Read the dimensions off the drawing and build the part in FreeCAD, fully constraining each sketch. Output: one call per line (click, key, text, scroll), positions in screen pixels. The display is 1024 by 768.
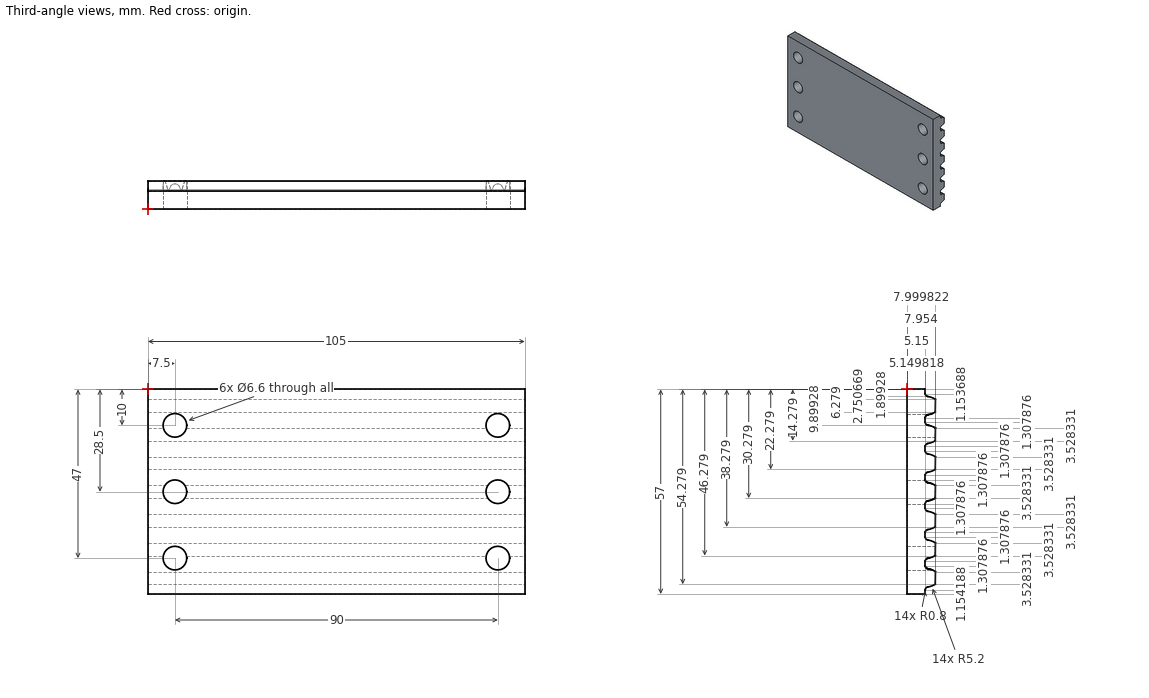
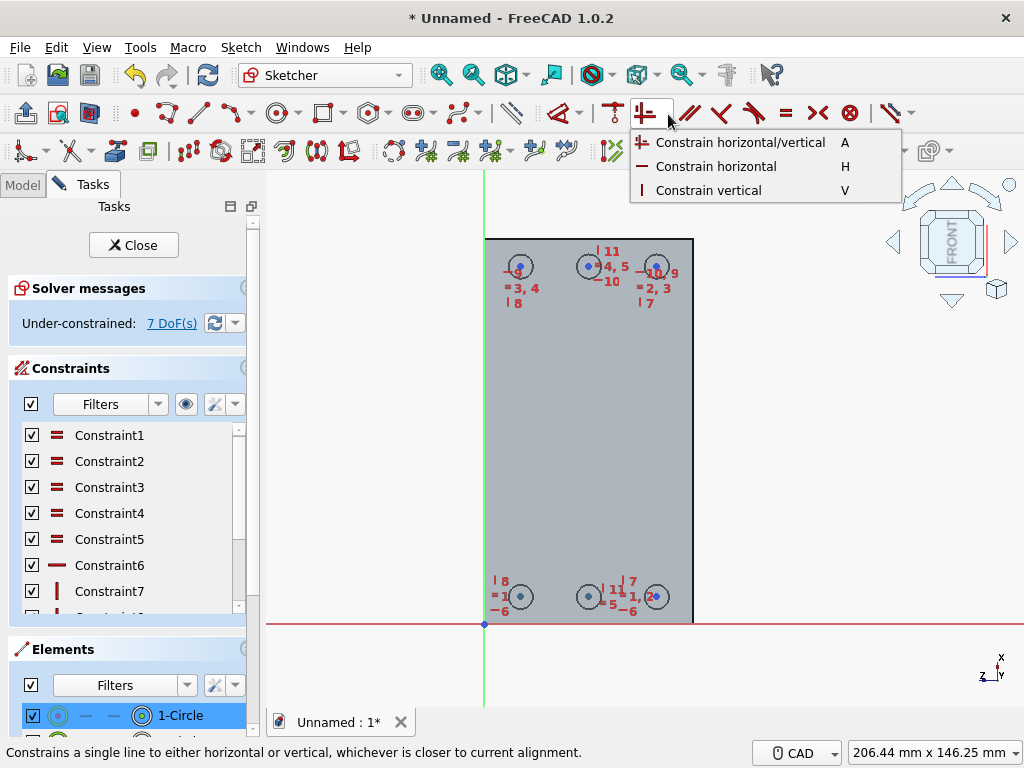
click(766, 166)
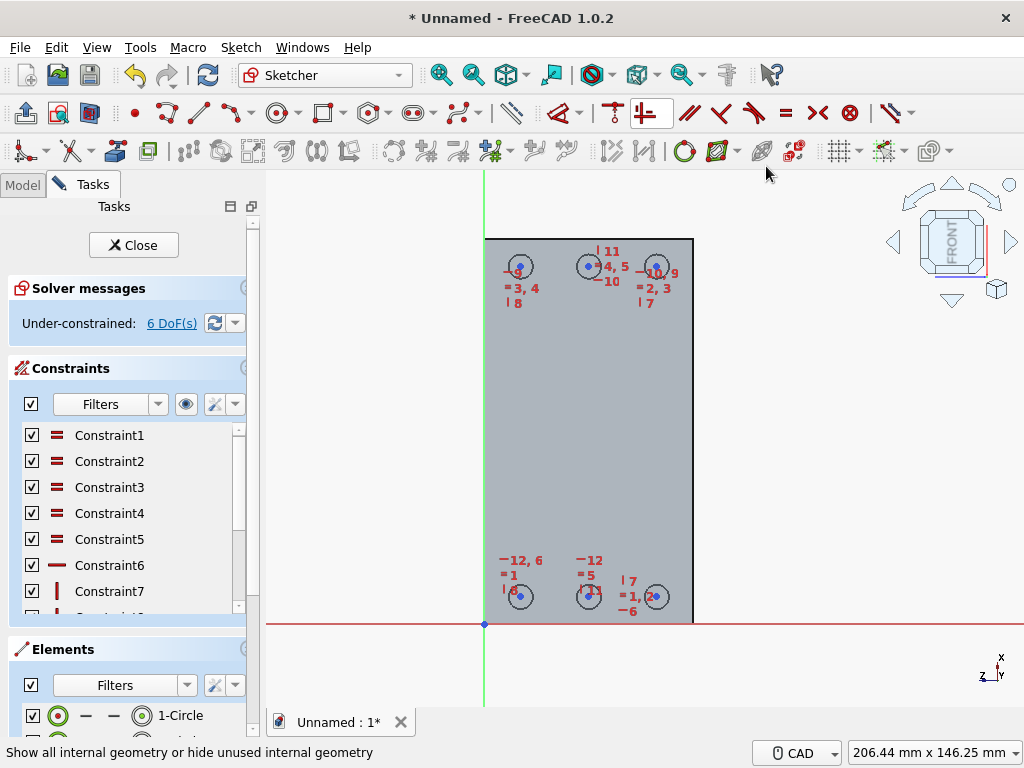
click(558, 114)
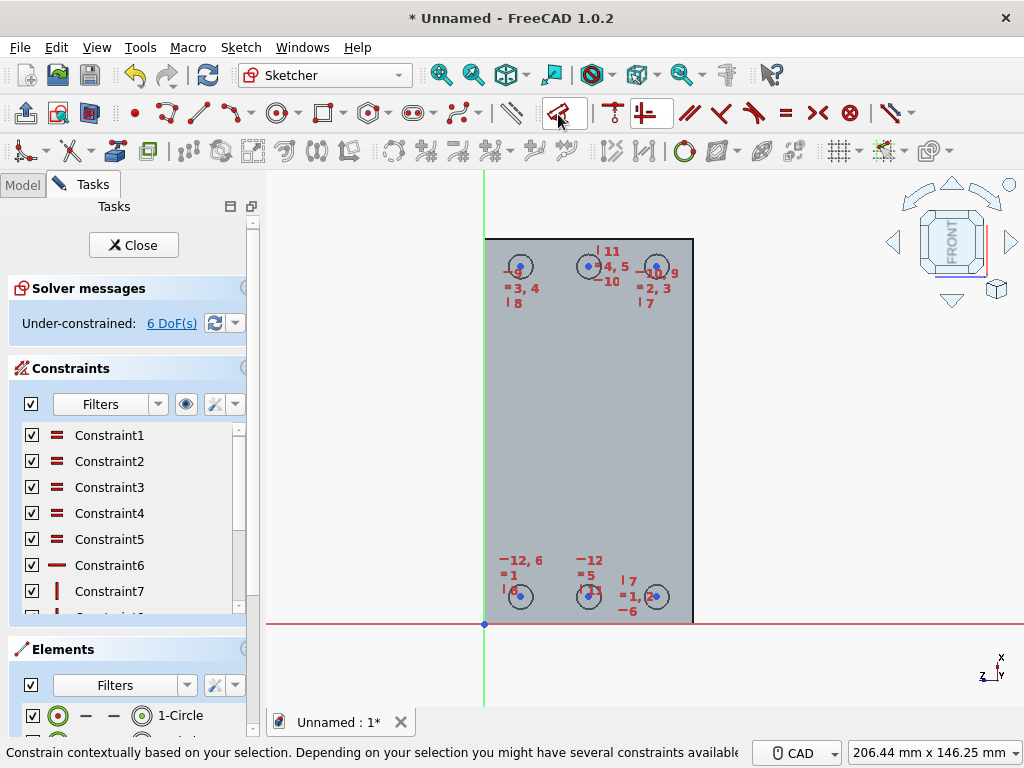
scroll(529, 588, up, 3)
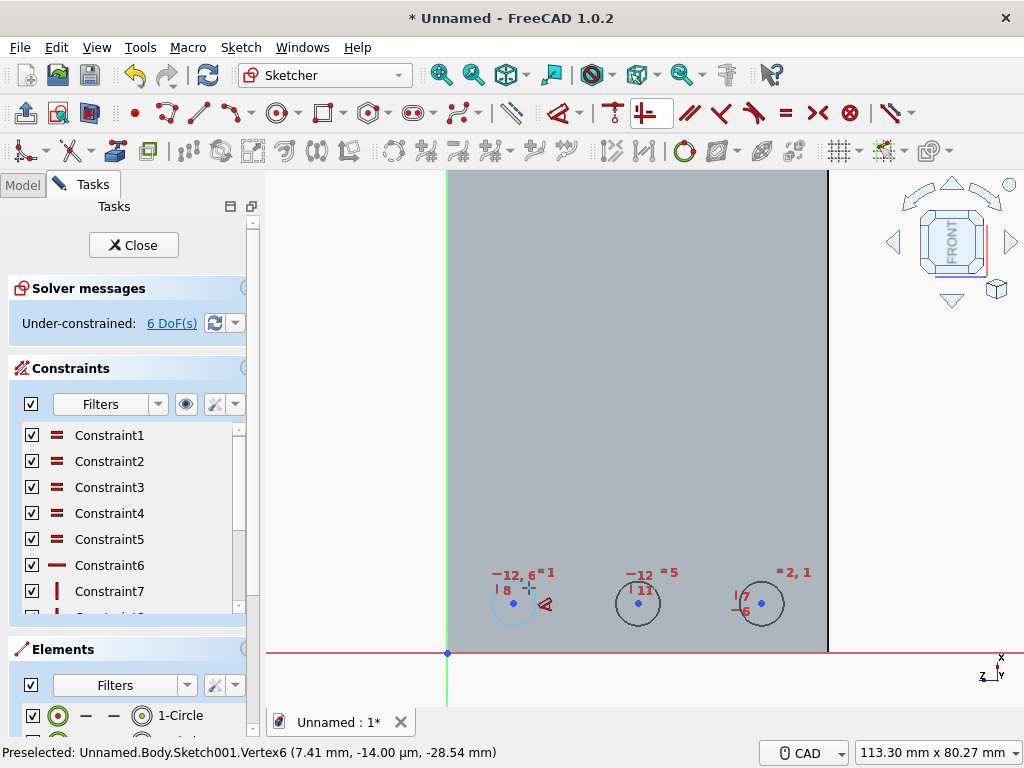
click(529, 588)
click(551, 565)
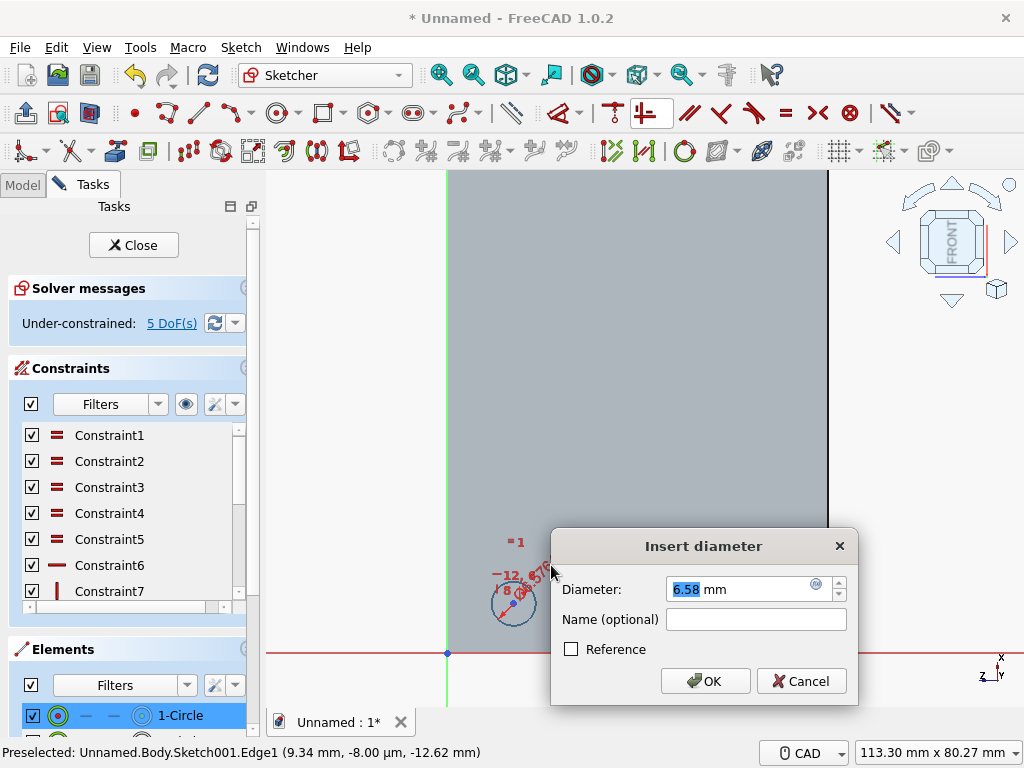
text(6.6)
key(Return)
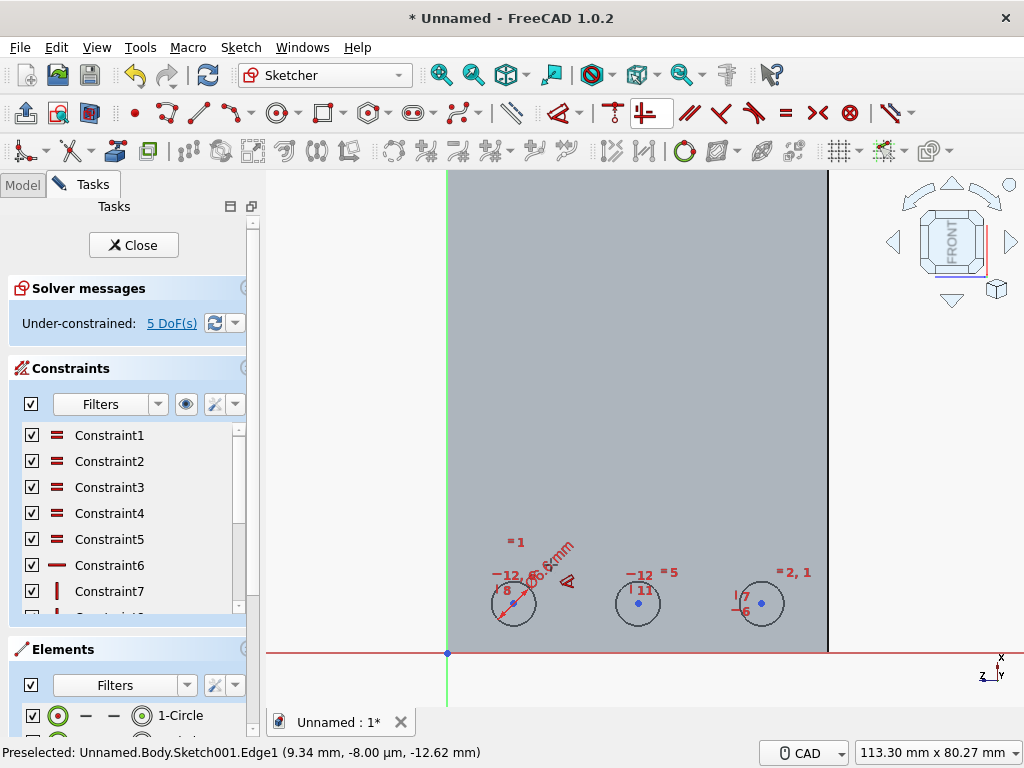
click(514, 604)
click(480, 570)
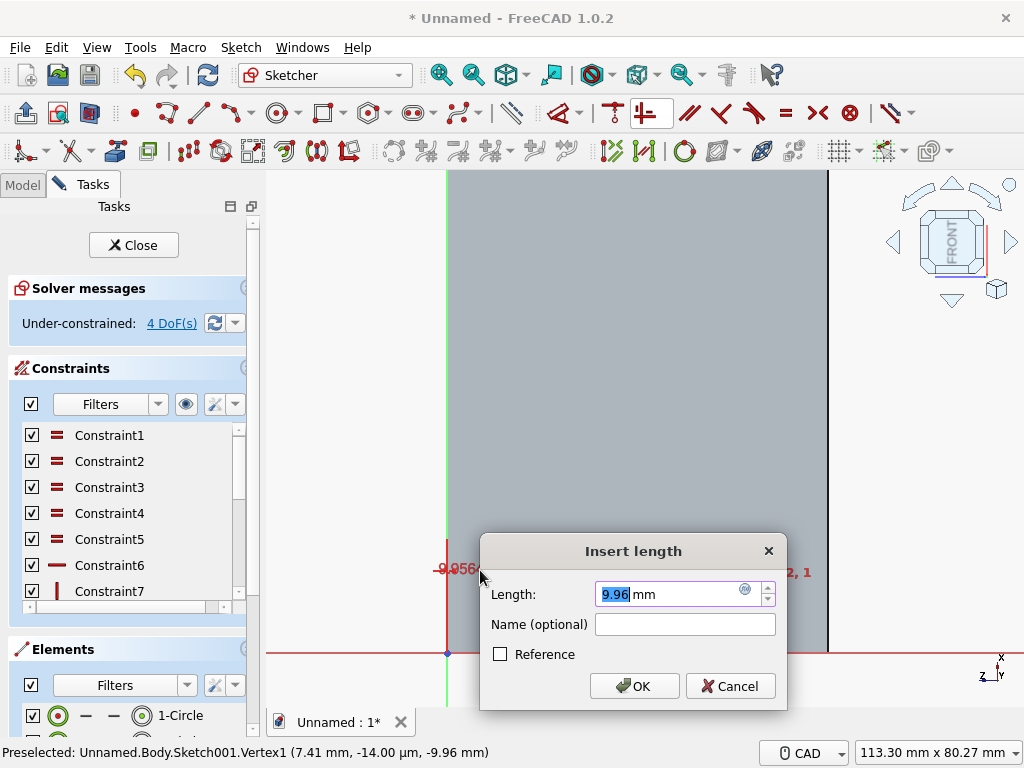
text(10)
key(Return)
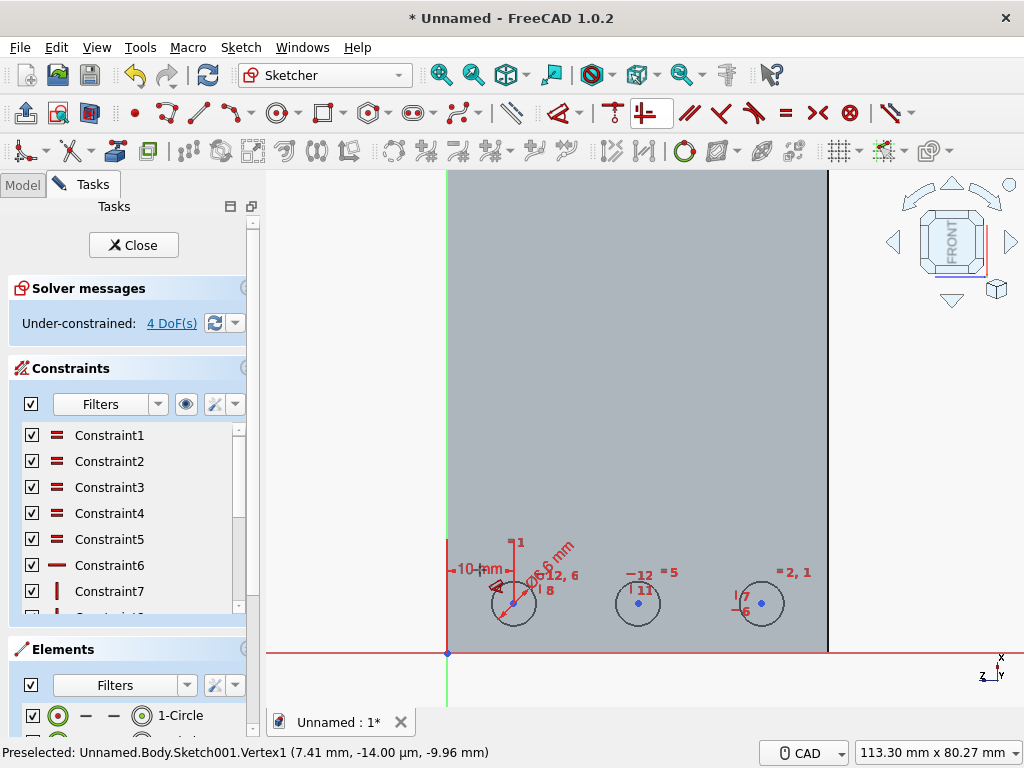
click(762, 604)
click(677, 570)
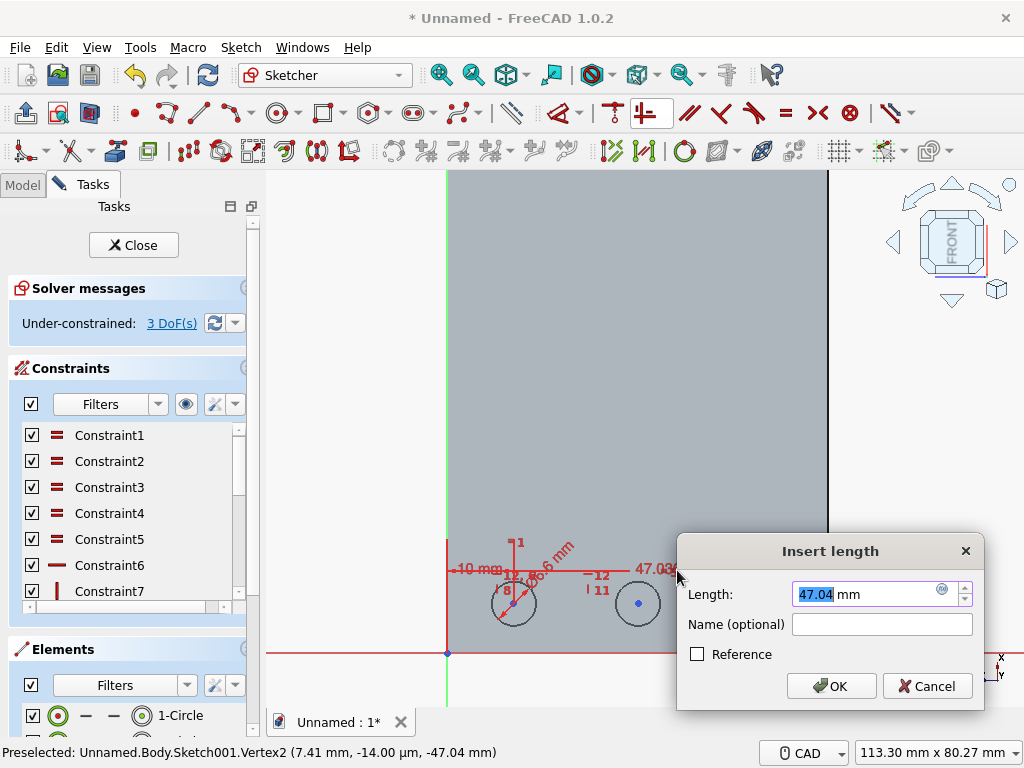
text(47)
key(Return)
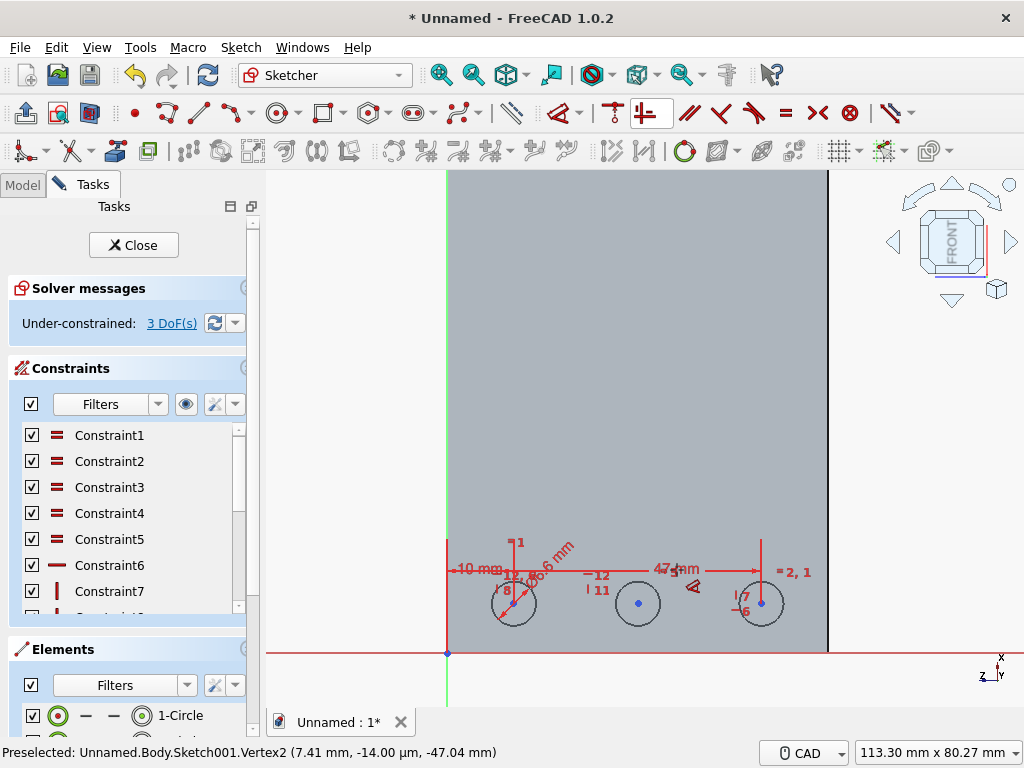
click(514, 604)
click(413, 629)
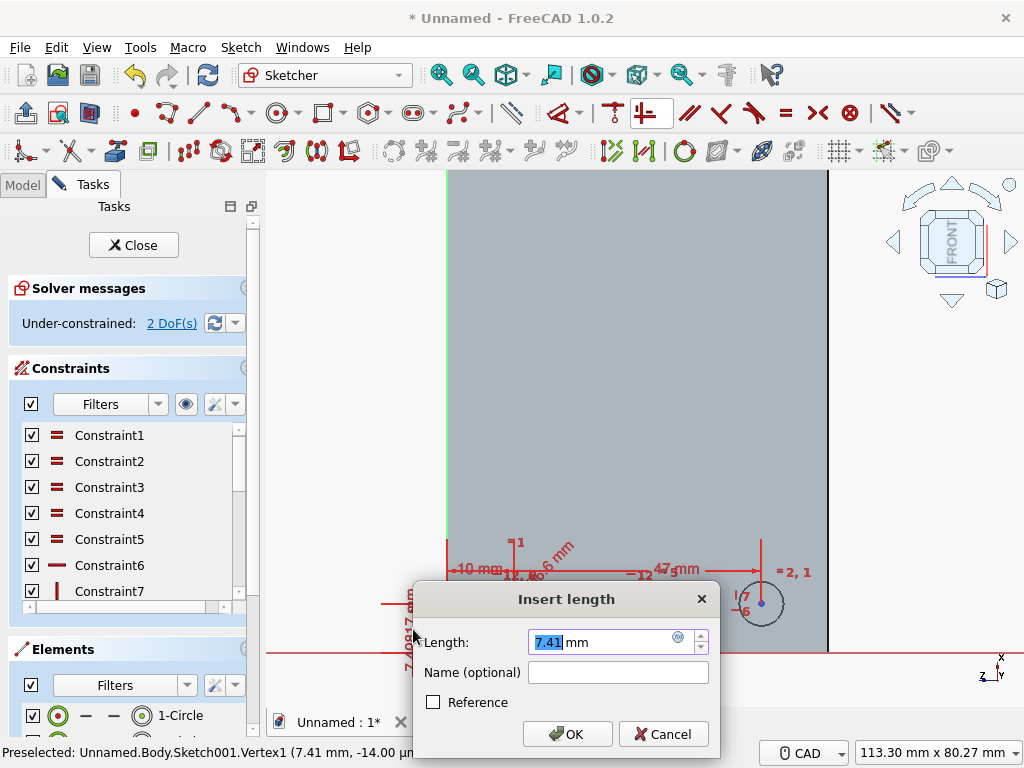
text(7.5)
key(Return)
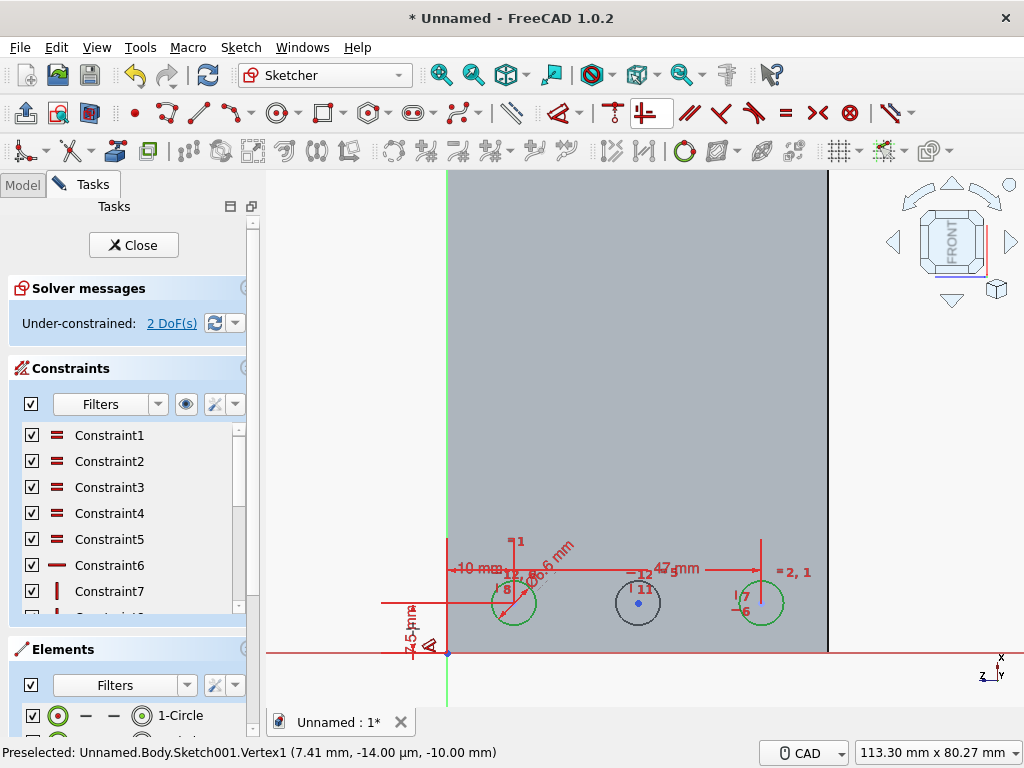
click(761, 603)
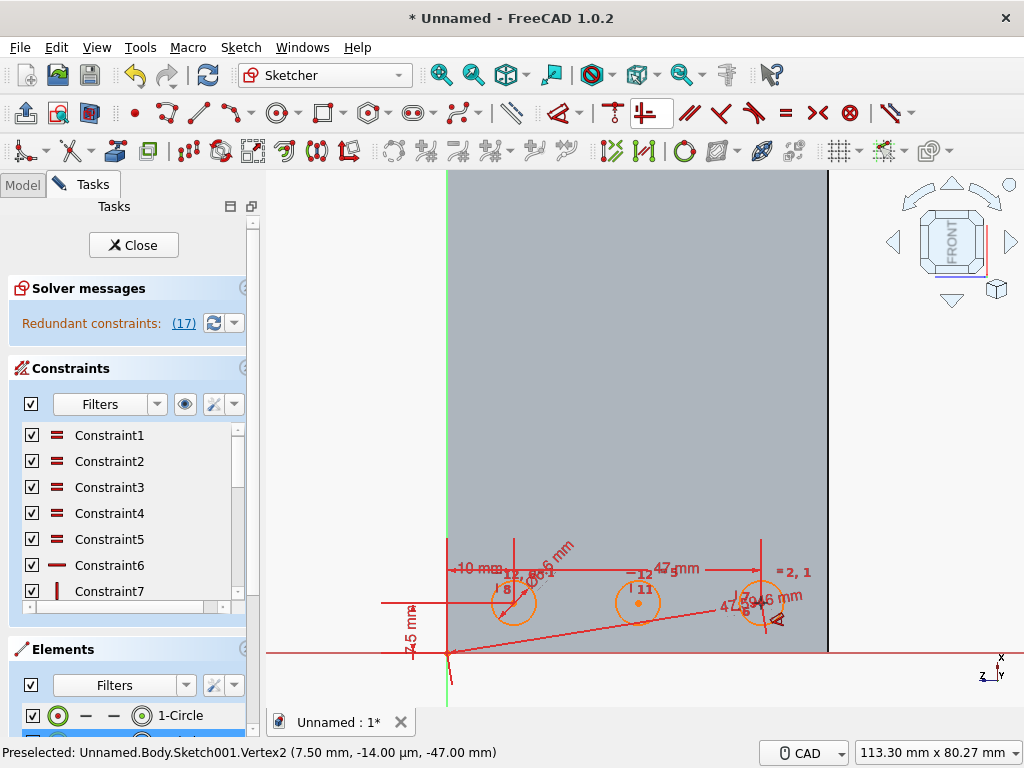
scroll(529, 587, down, 3)